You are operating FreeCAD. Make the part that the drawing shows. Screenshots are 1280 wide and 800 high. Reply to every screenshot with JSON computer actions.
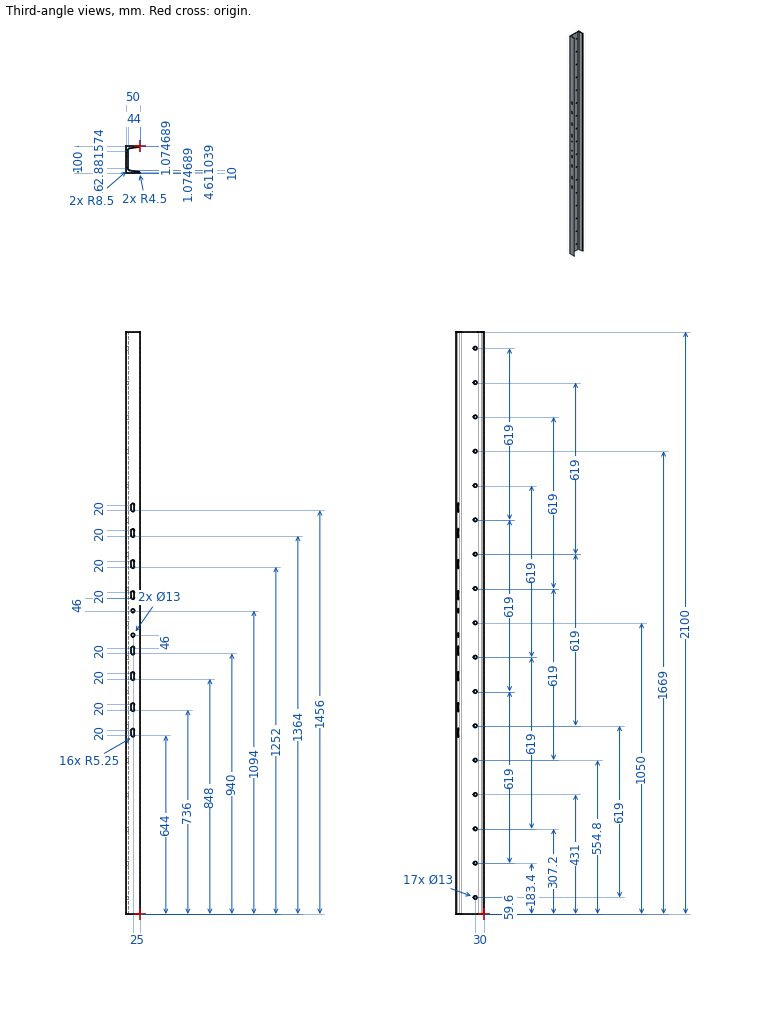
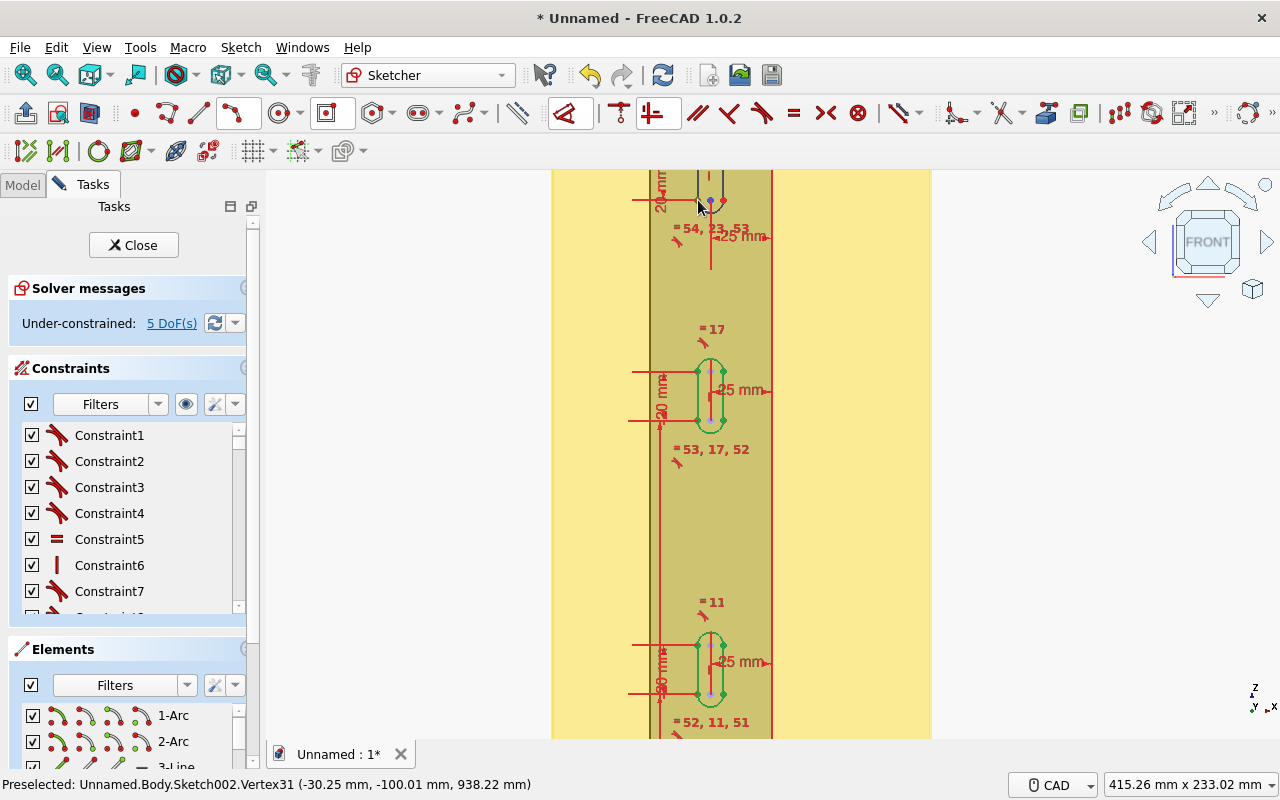
{"action": "key", "text": "i"}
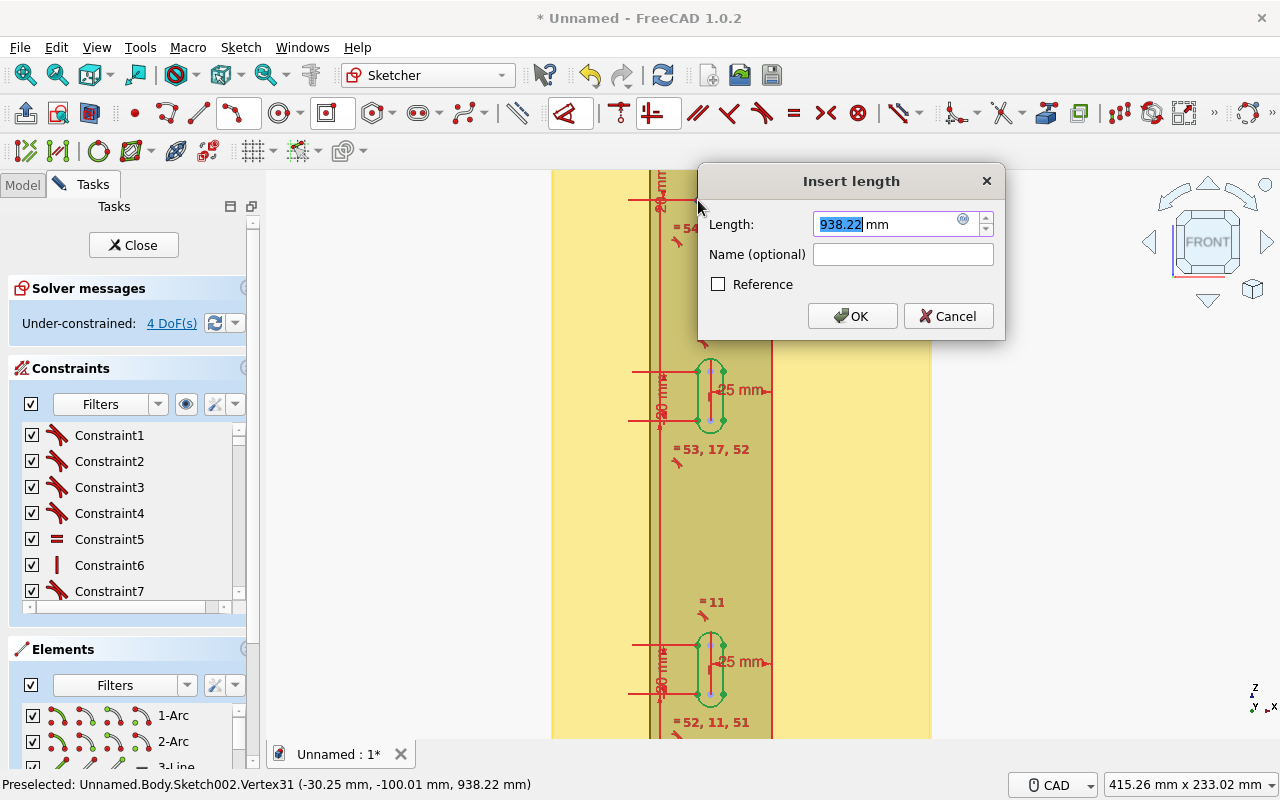
{"action": "type", "text": "940"}
{"action": "key", "text": "Return"}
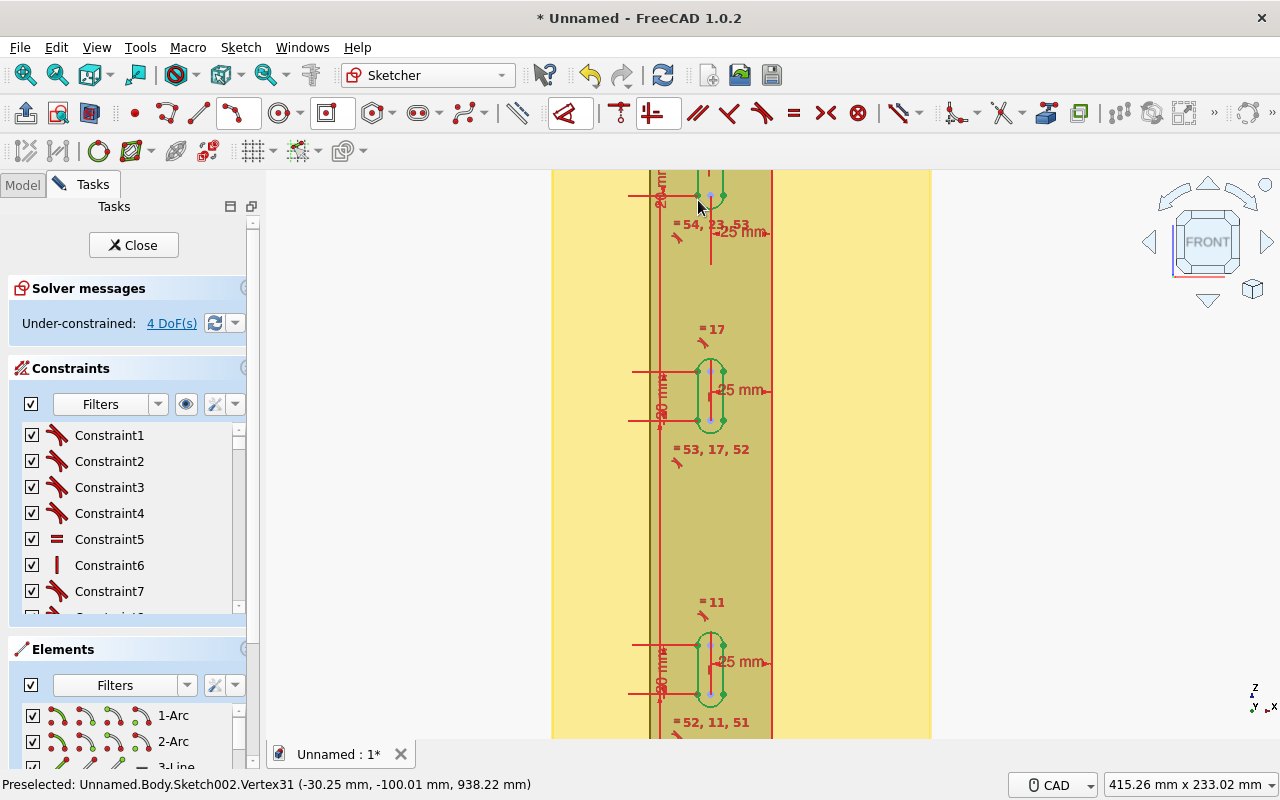
{"action": "scroll", "coordinate": [702, 432], "scroll_direction": "down", "scroll_amount": 12}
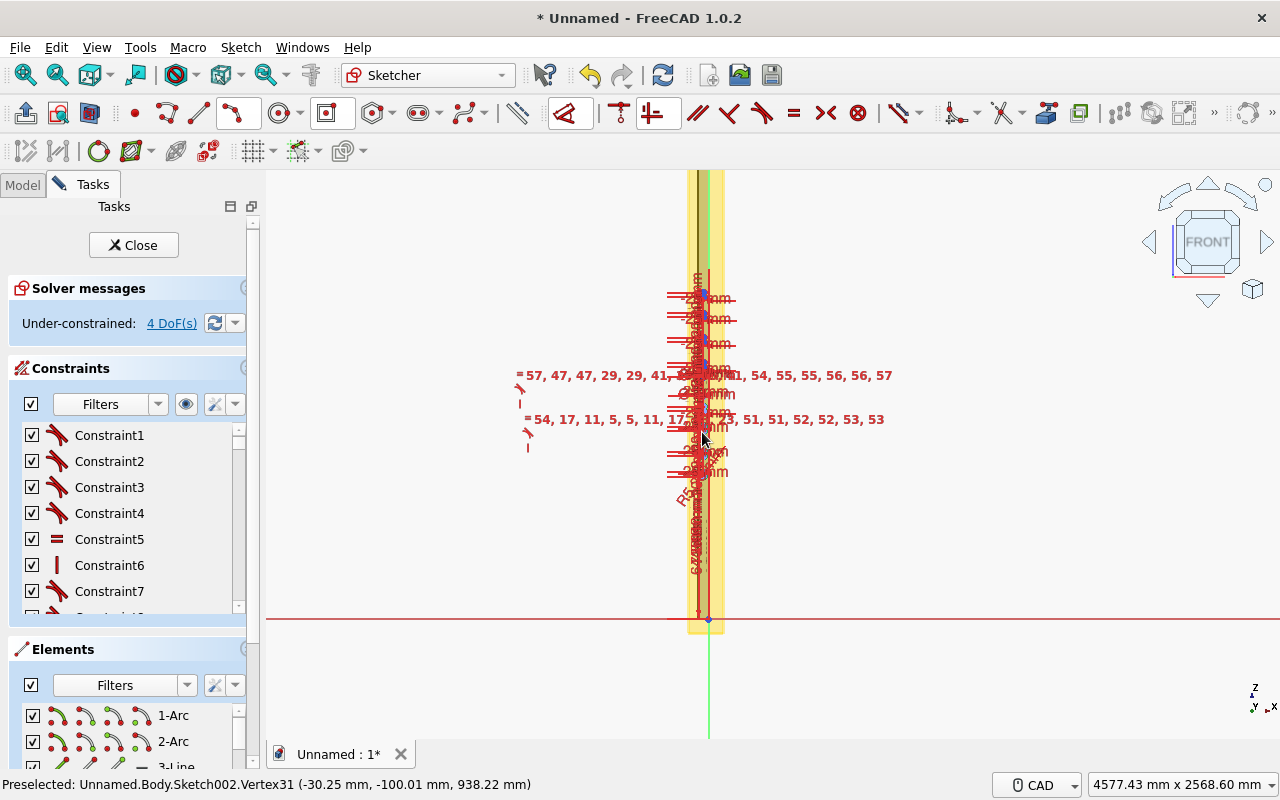
{"action": "scroll", "coordinate": [703, 377], "scroll_direction": "up", "scroll_amount": 4}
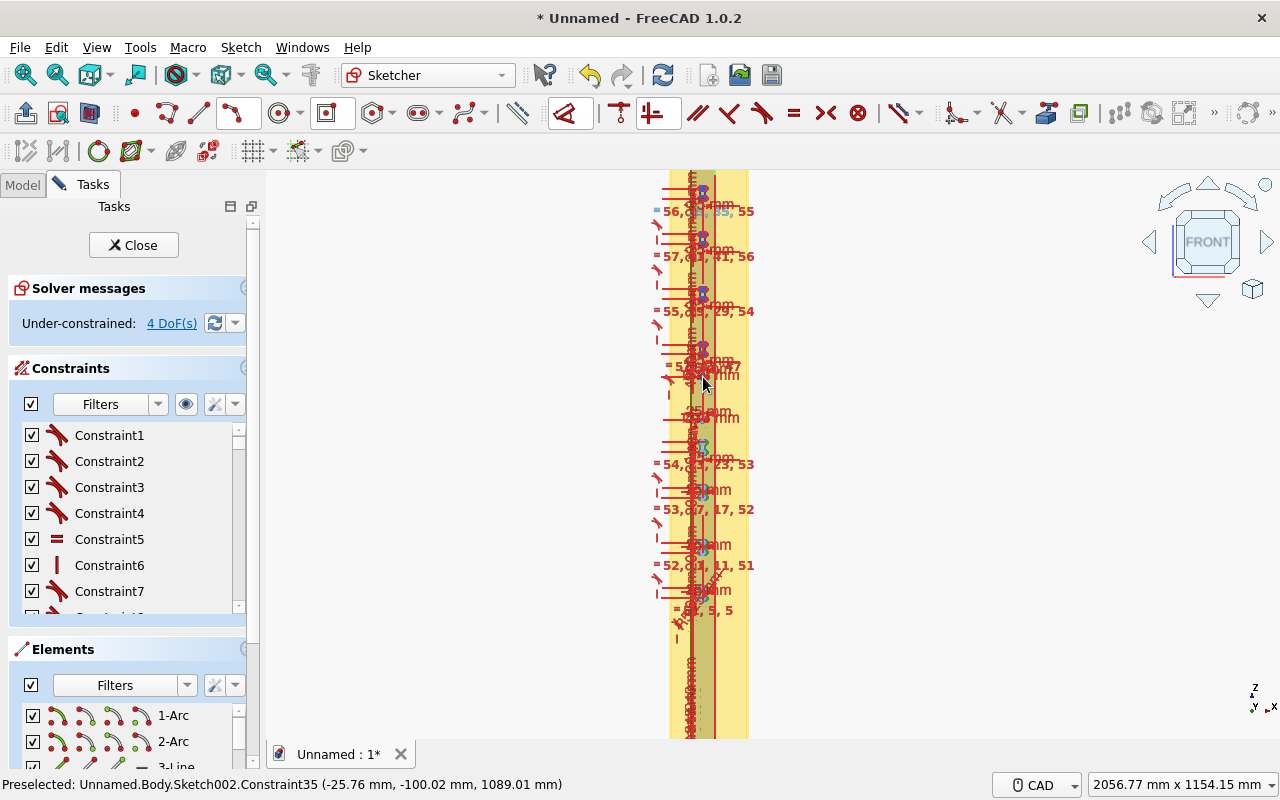
{"action": "scroll", "coordinate": [703, 377], "scroll_direction": "up", "scroll_amount": 4}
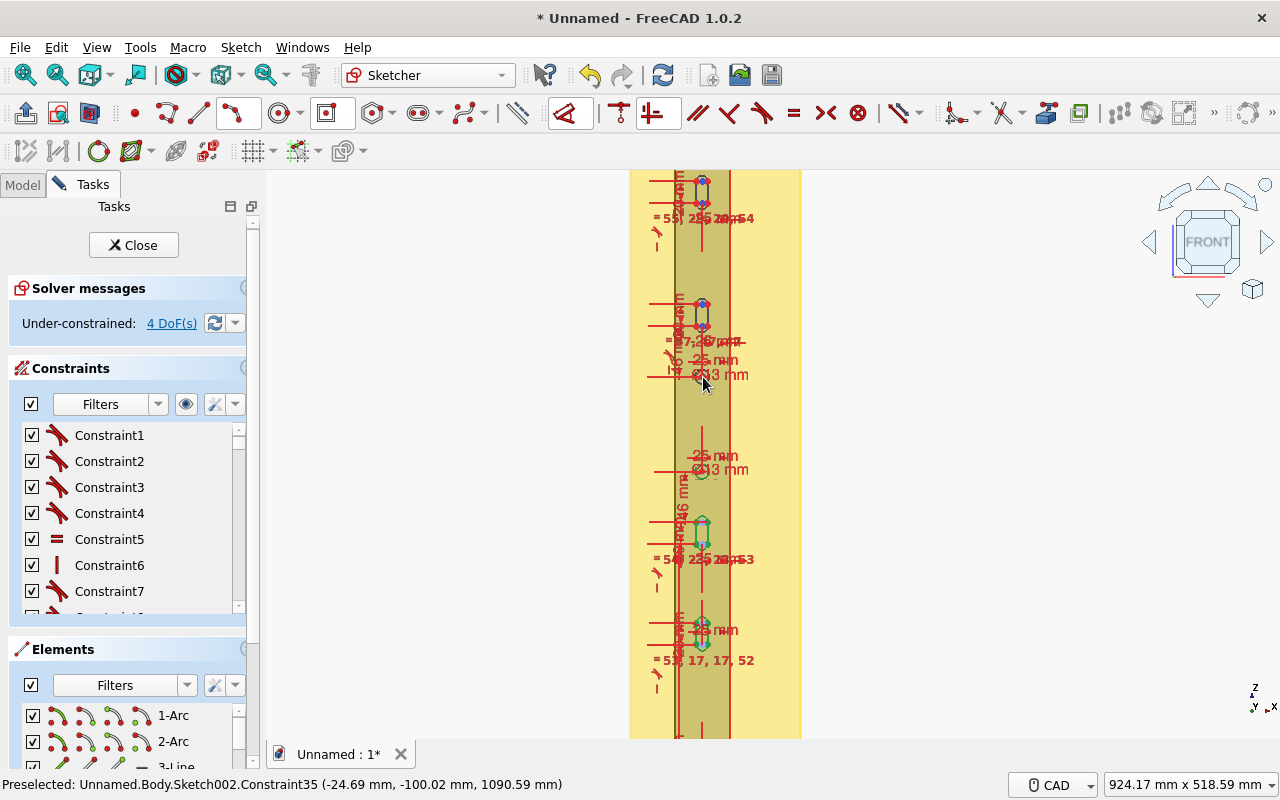
{"action": "left_click", "coordinate": [702, 377]}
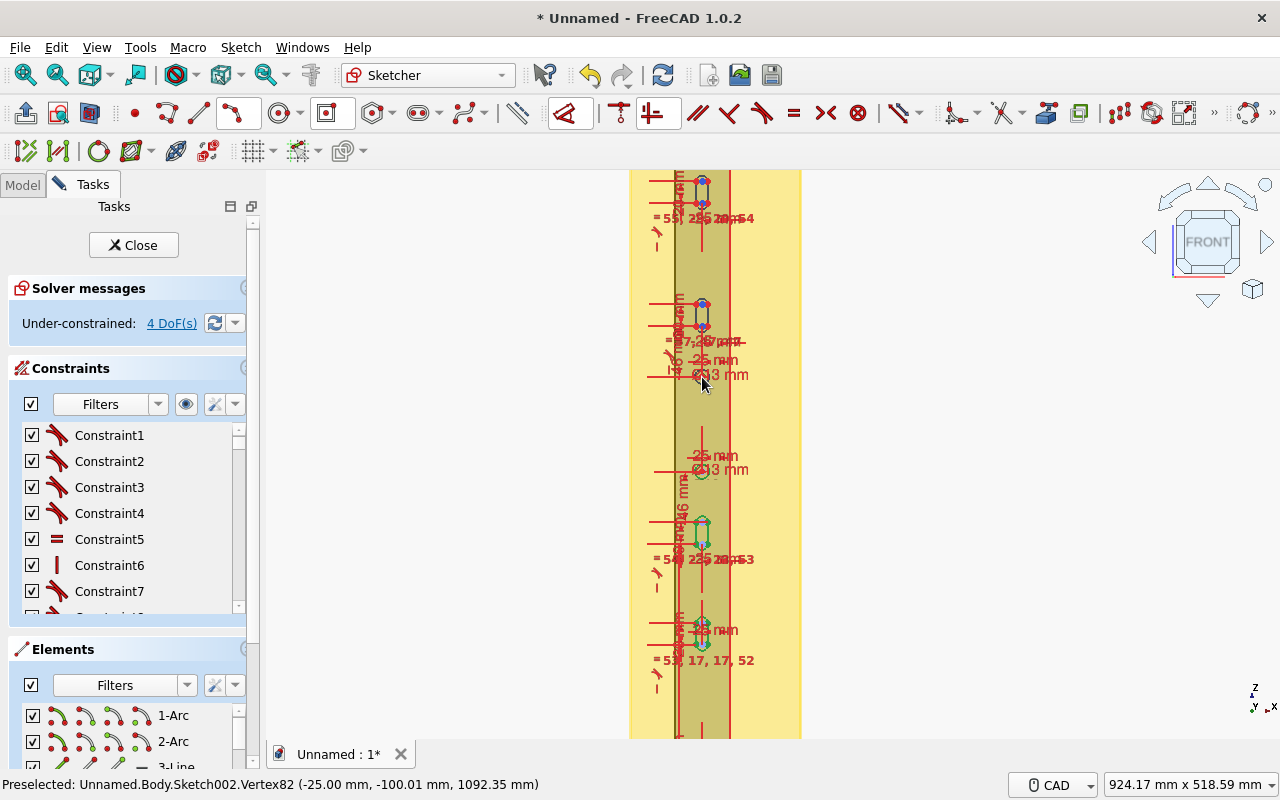
{"action": "key", "text": "i"}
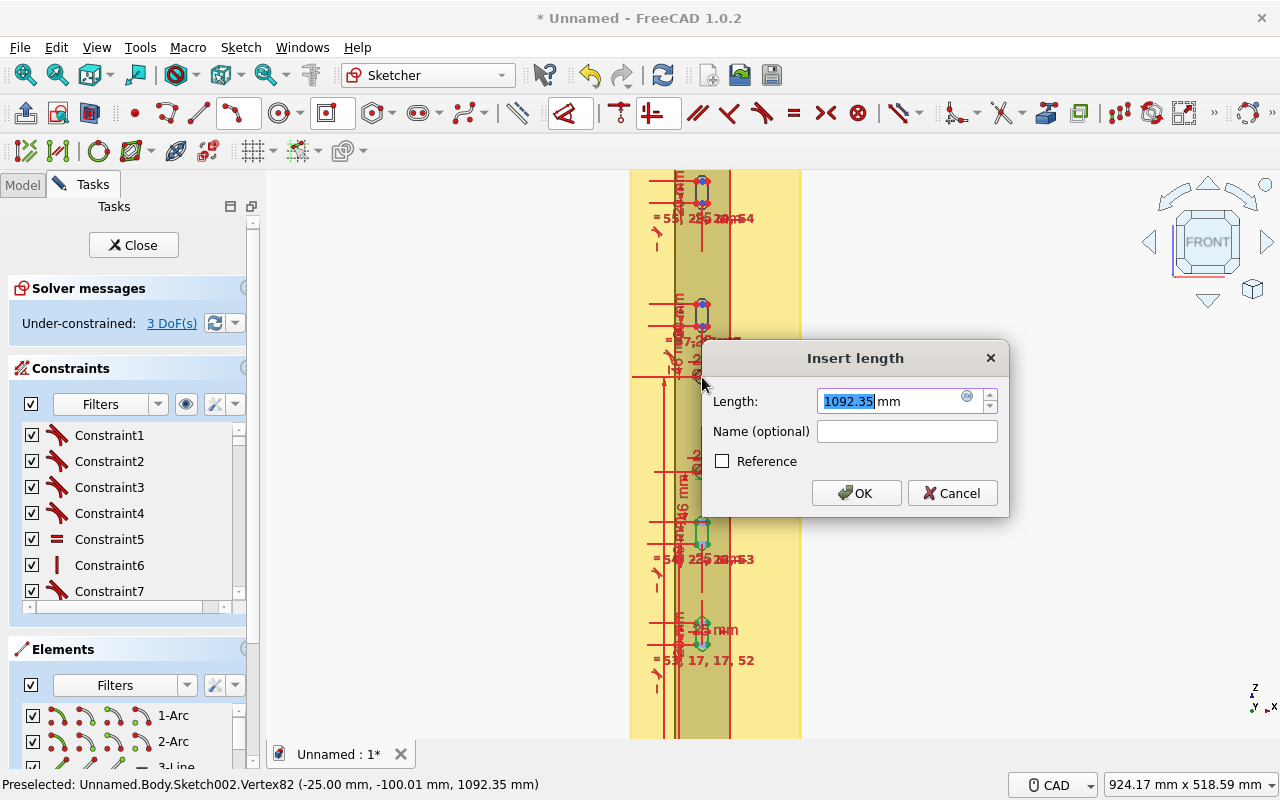
{"action": "type", "text": "1094"}
{"action": "key", "text": "Return"}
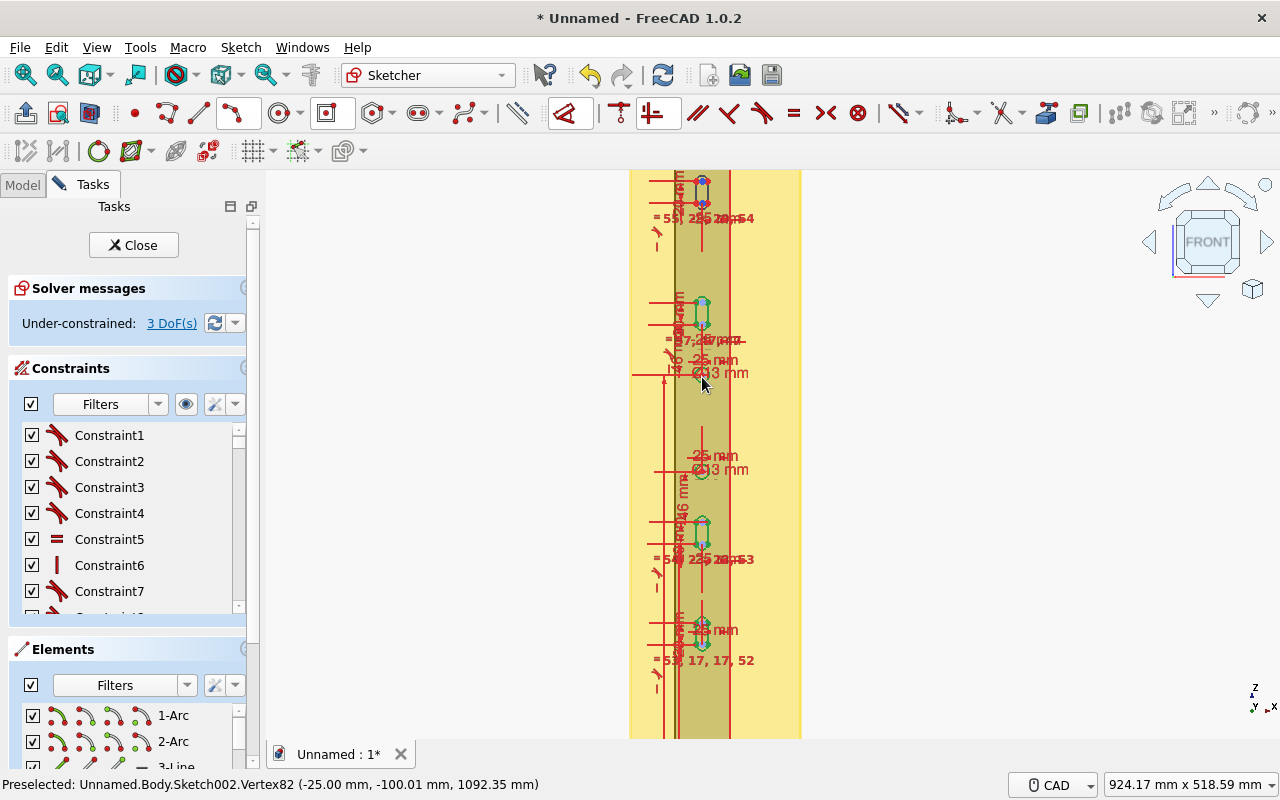
{"action": "scroll", "coordinate": [696, 203], "scroll_direction": "up", "scroll_amount": 4}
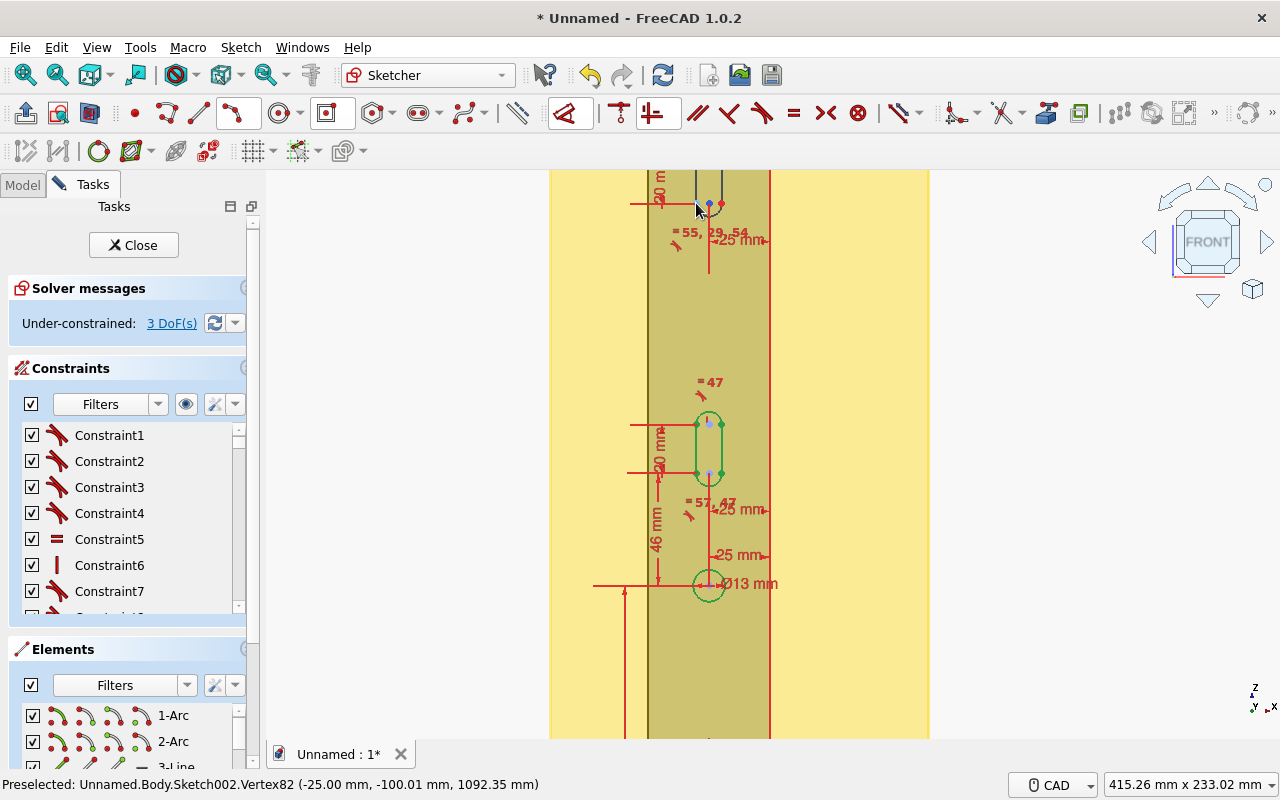
{"action": "left_click", "coordinate": [696, 204]}